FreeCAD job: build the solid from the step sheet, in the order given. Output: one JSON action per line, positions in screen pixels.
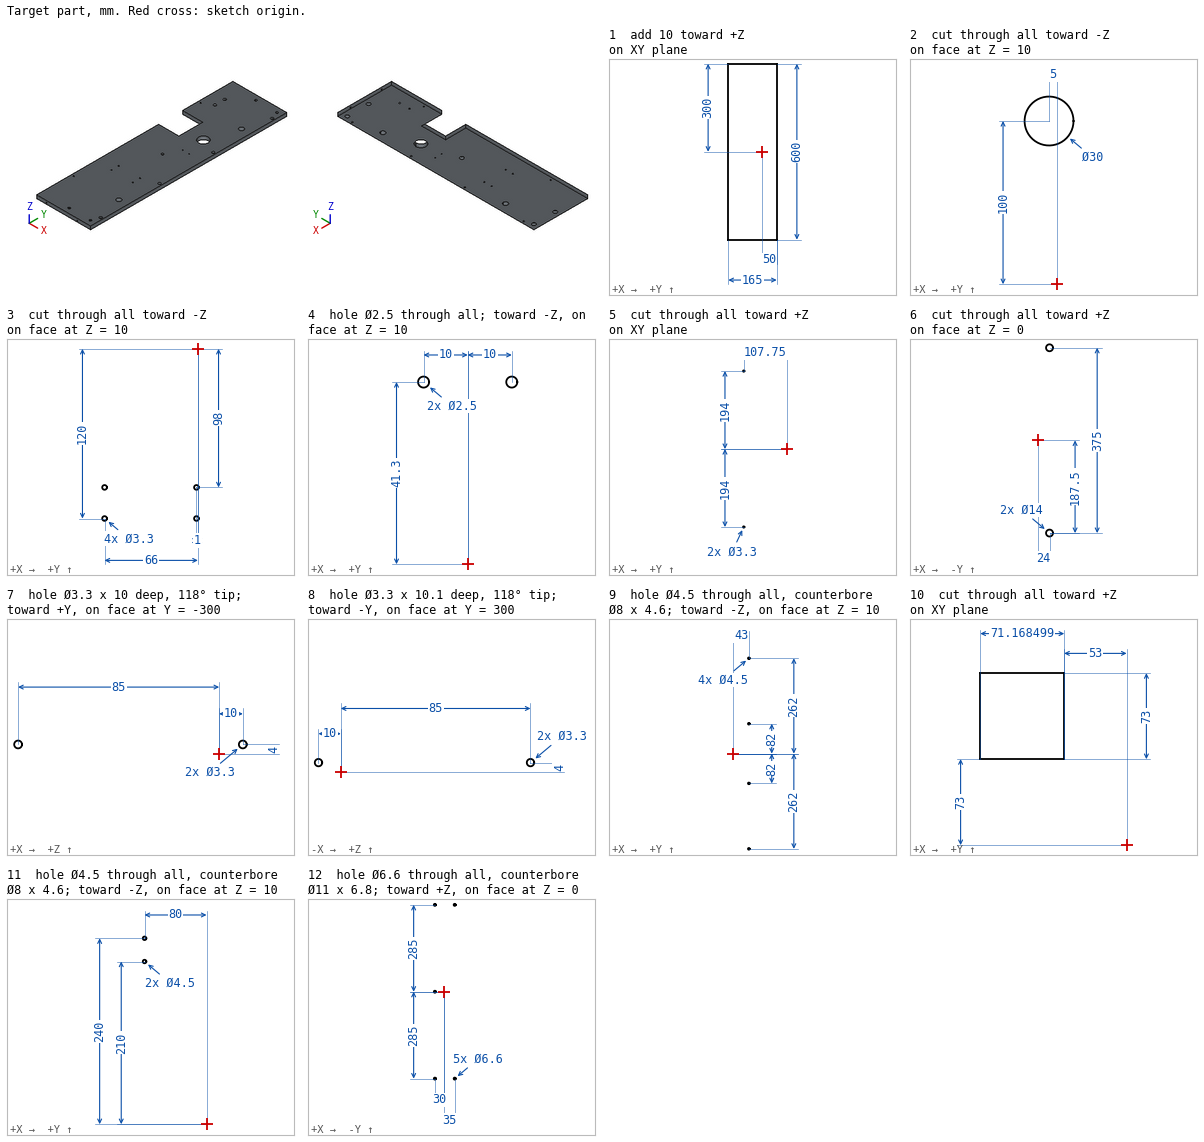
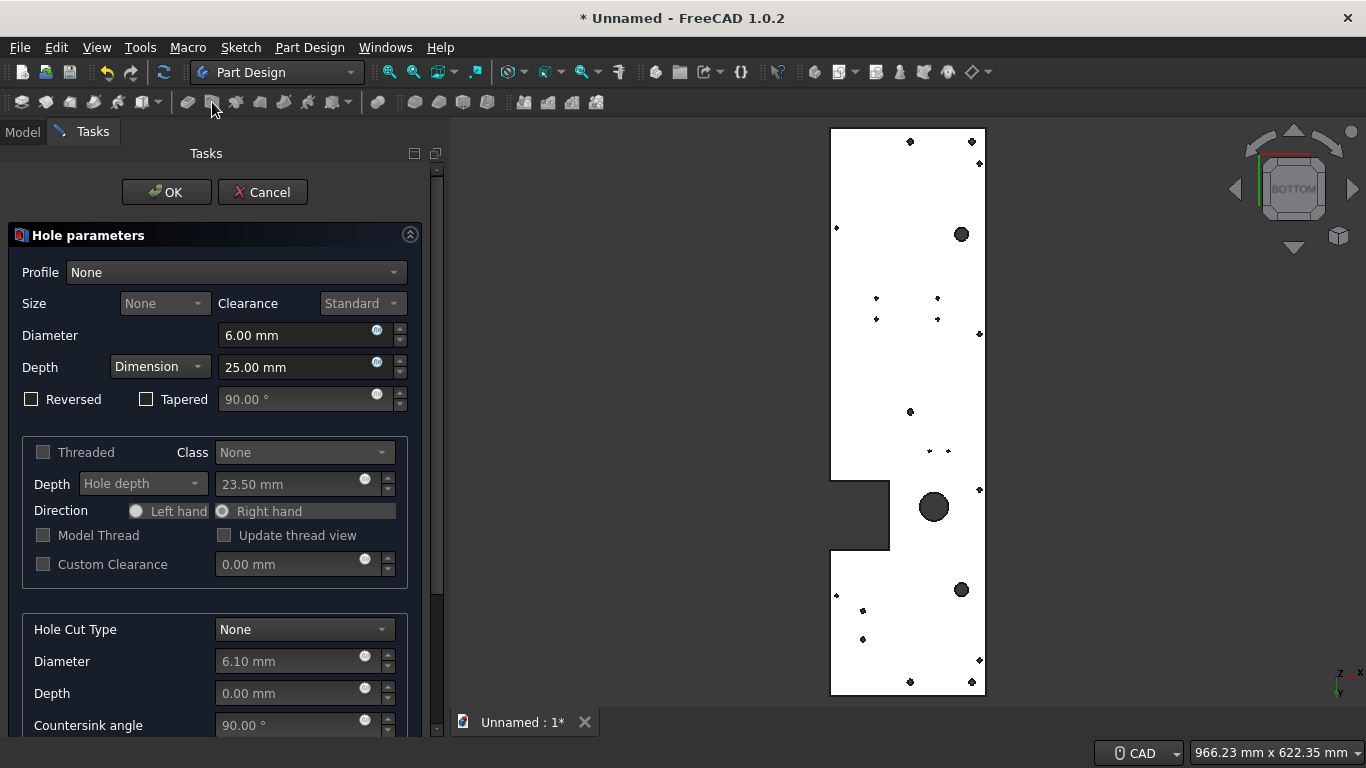
{"action": "triple_click", "coordinate": [305, 335]}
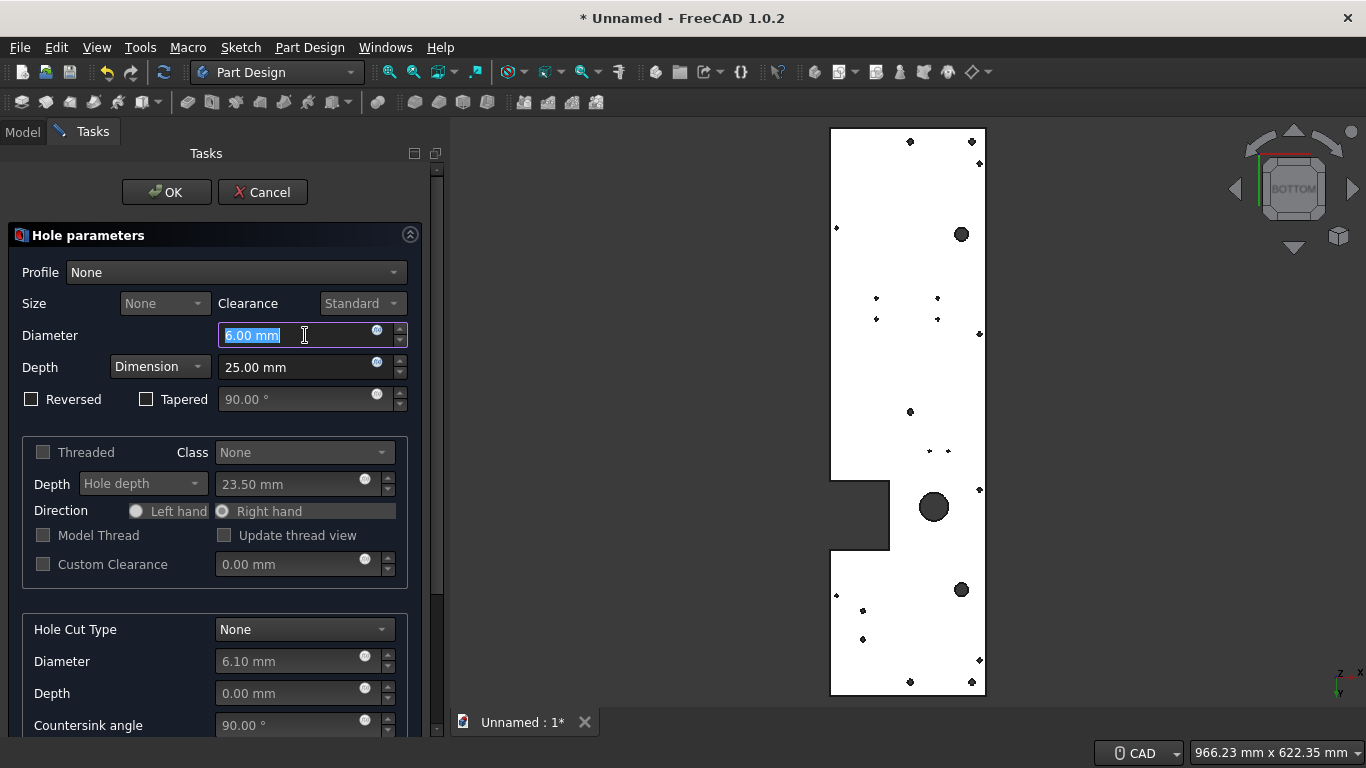
{"action": "type", "text": "6.6"}
{"action": "key", "text": "Tab"}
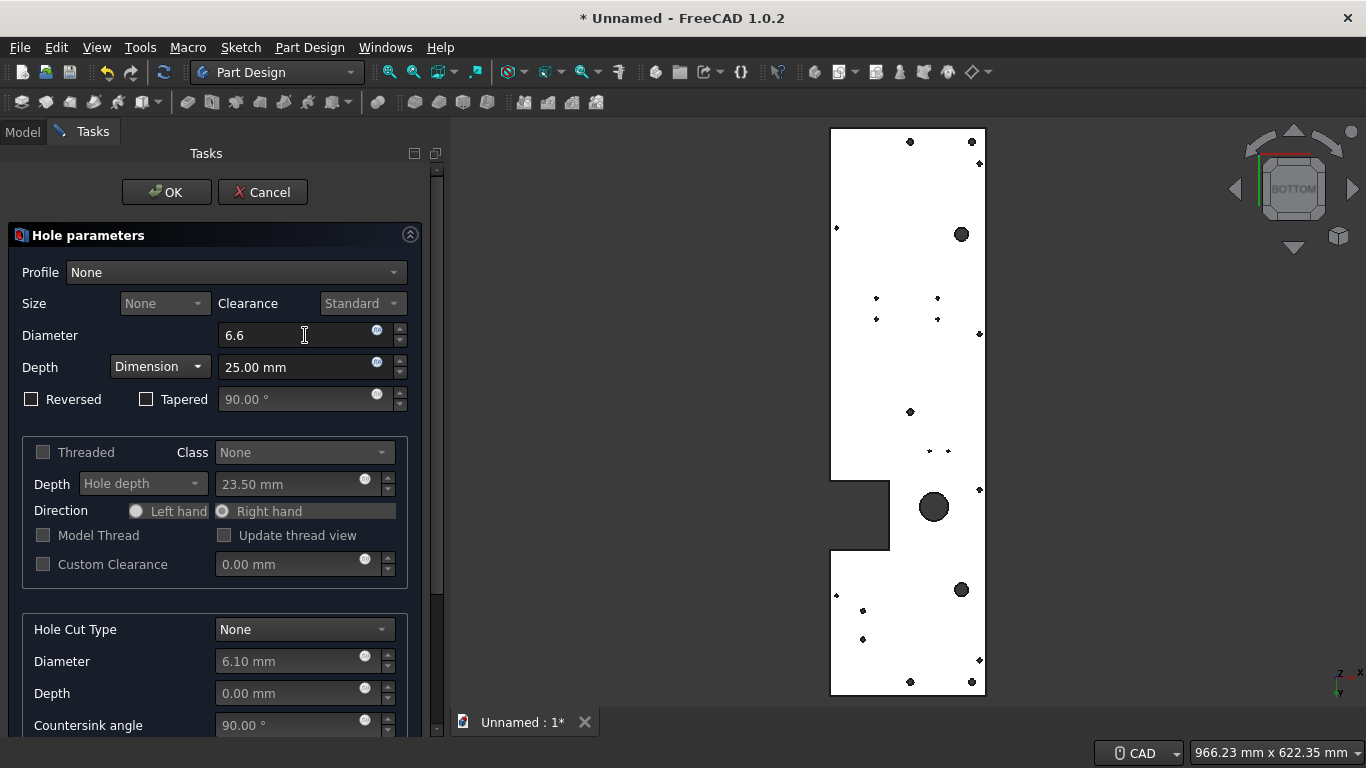
{"action": "left_click", "coordinate": [161, 366]}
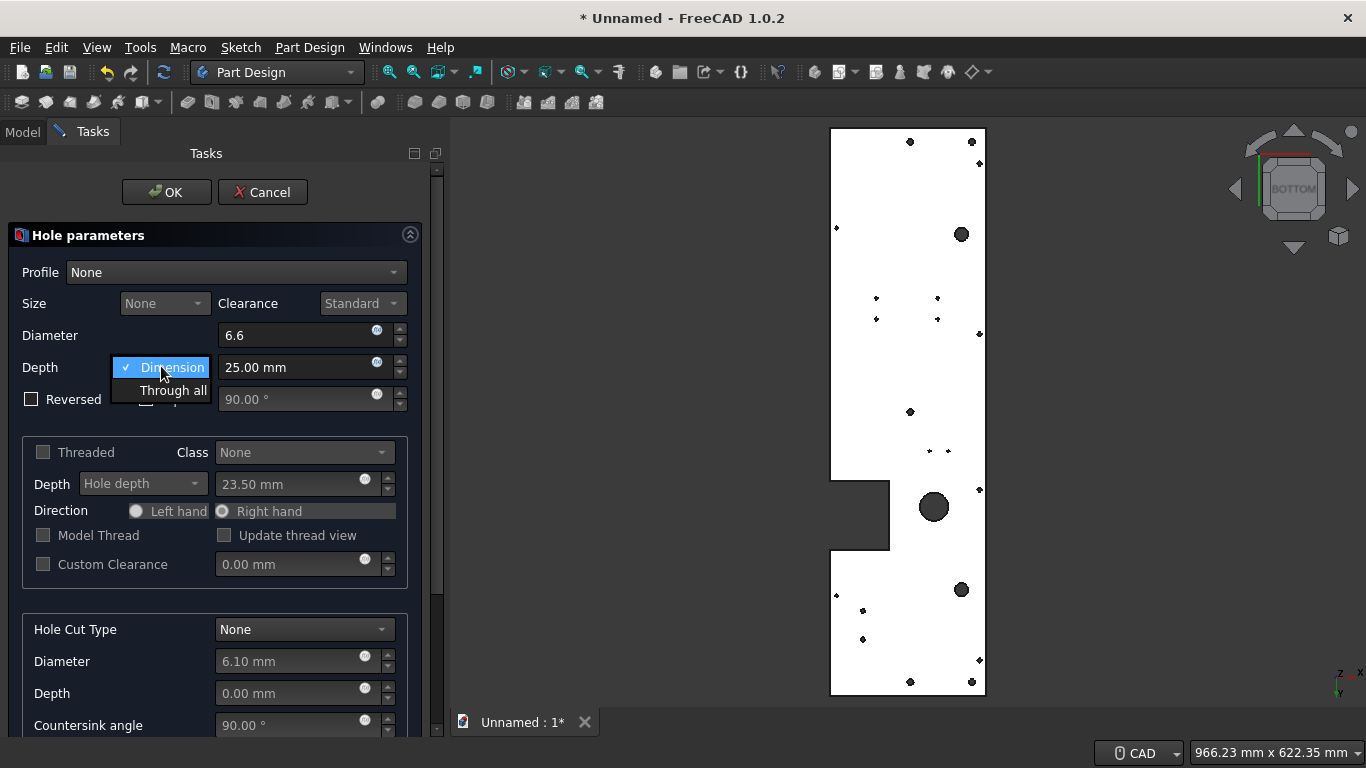
{"action": "left_click", "coordinate": [160, 390]}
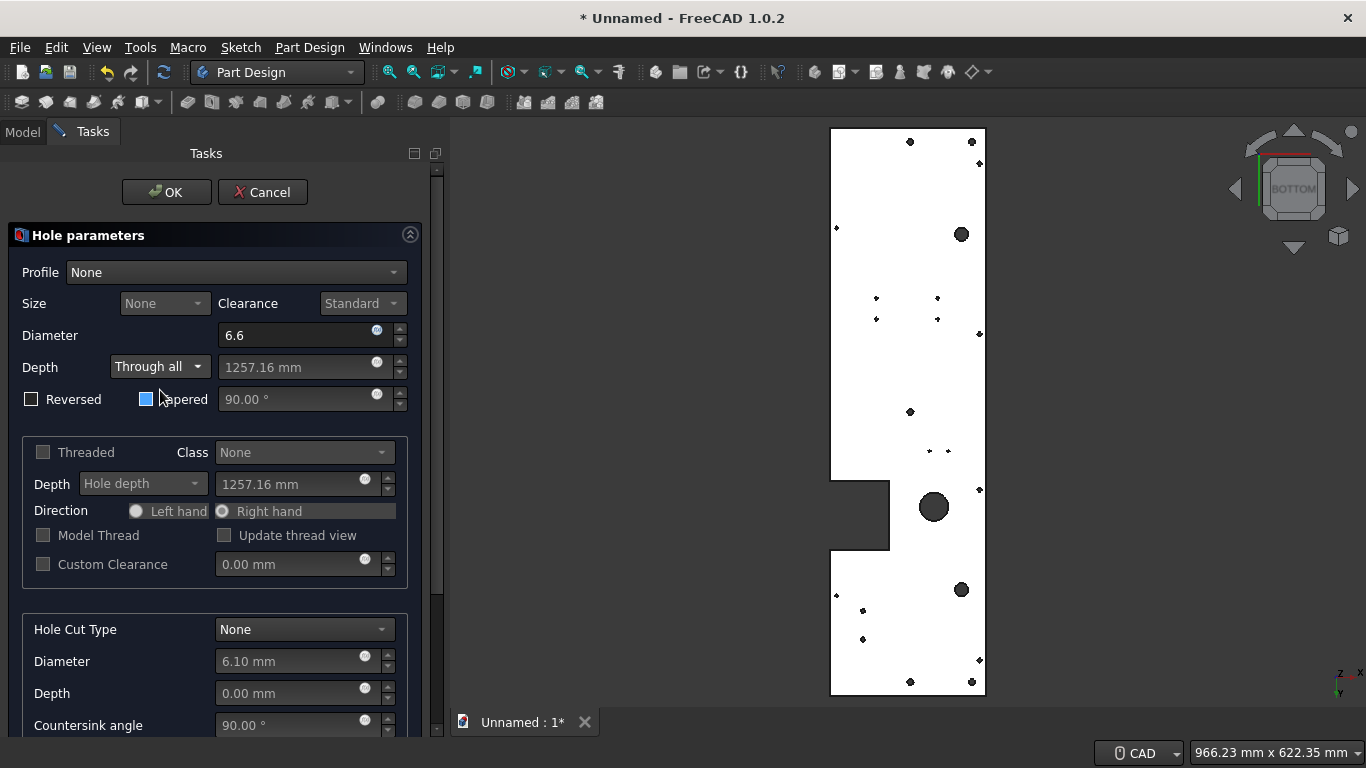
{"action": "left_click", "coordinate": [306, 630]}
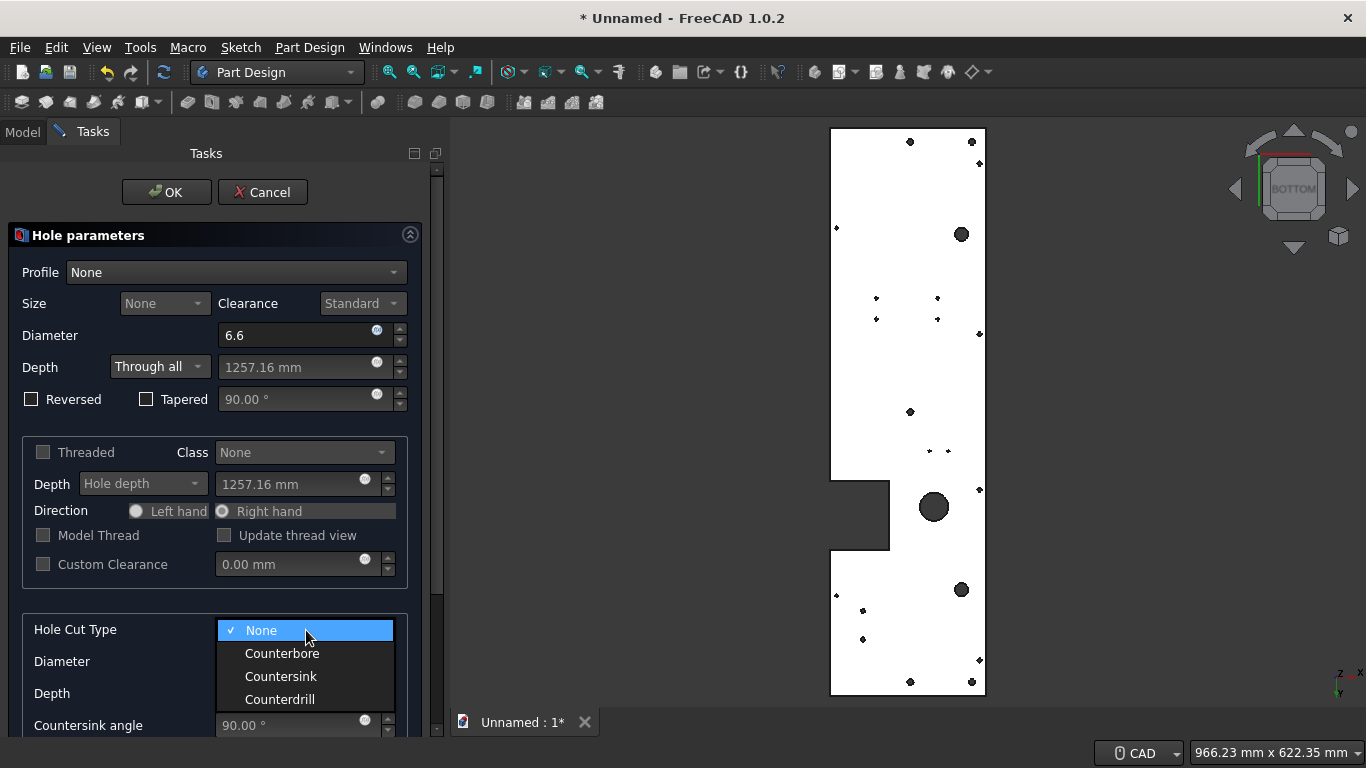
{"action": "left_click", "coordinate": [304, 654]}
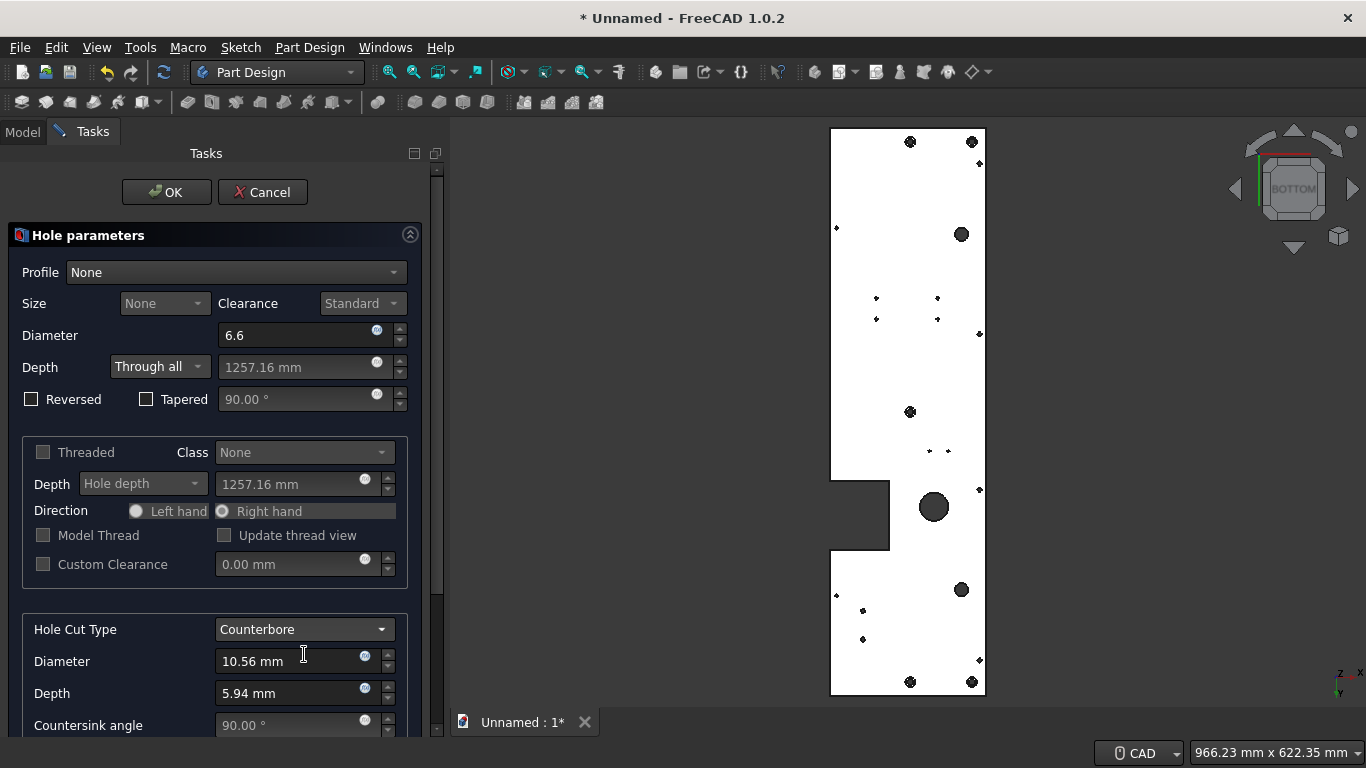
{"action": "triple_click", "coordinate": [298, 661]}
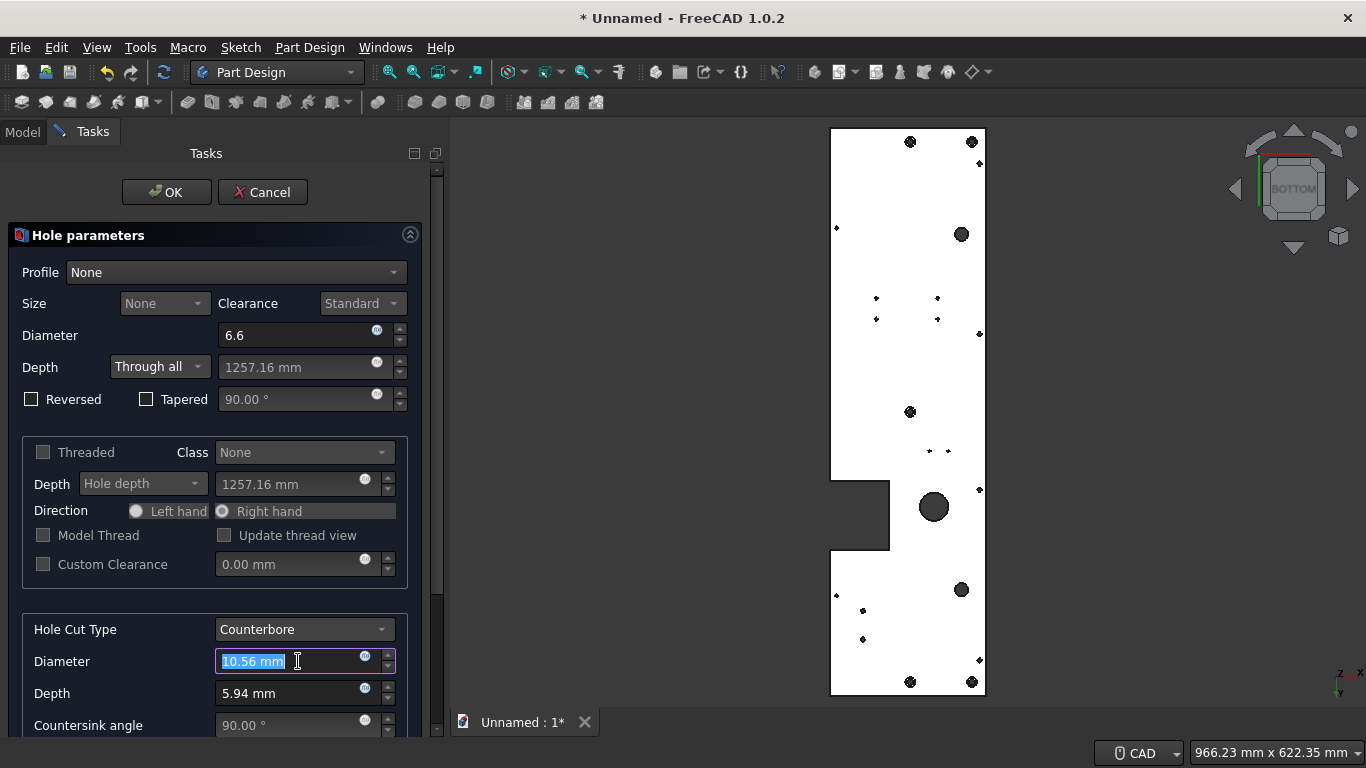
{"action": "type", "text": "11"}
{"action": "key", "text": "Tab"}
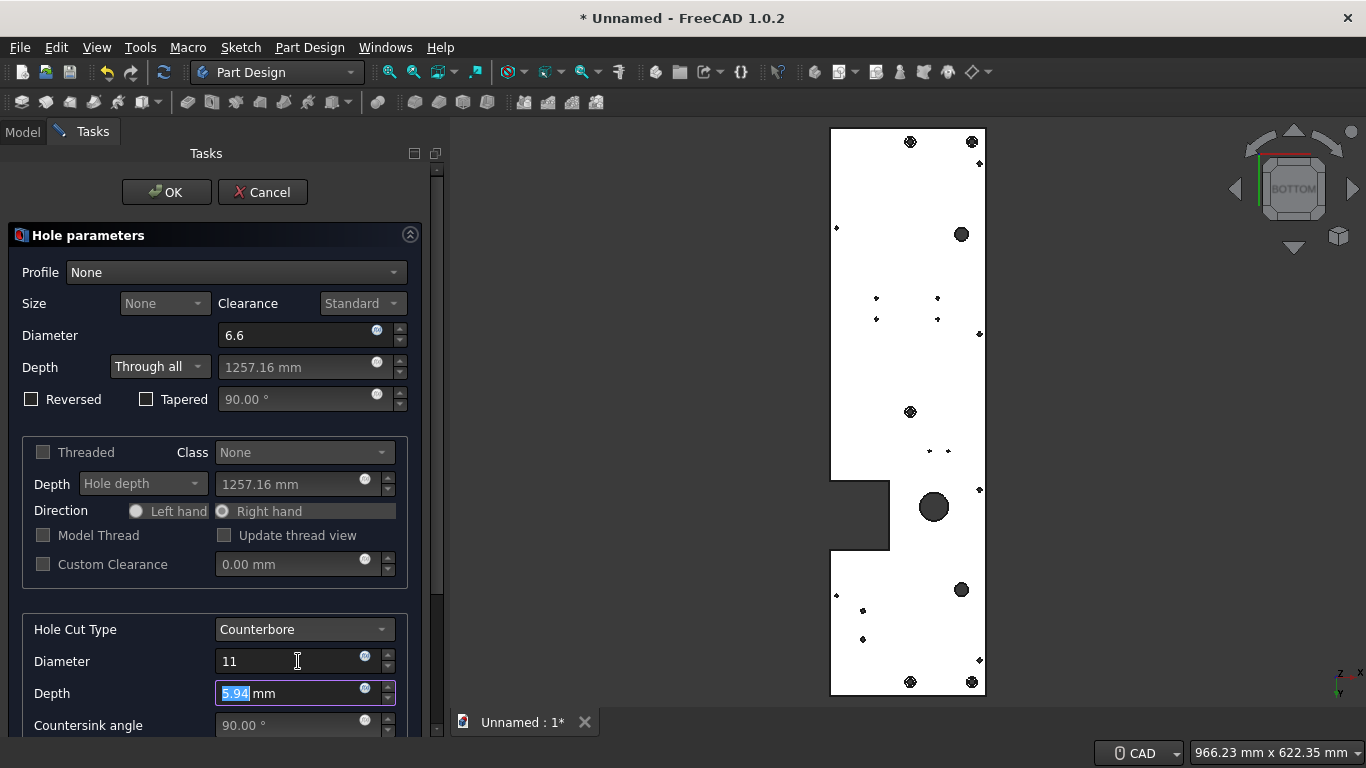
{"action": "type", "text": "6.8"}
{"action": "key", "text": "Tab"}